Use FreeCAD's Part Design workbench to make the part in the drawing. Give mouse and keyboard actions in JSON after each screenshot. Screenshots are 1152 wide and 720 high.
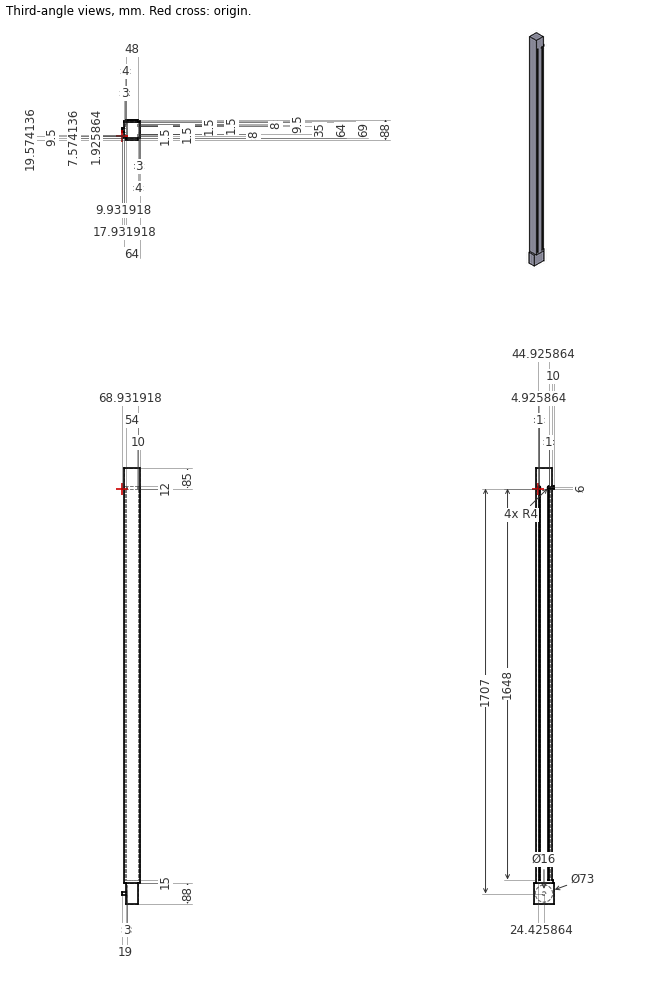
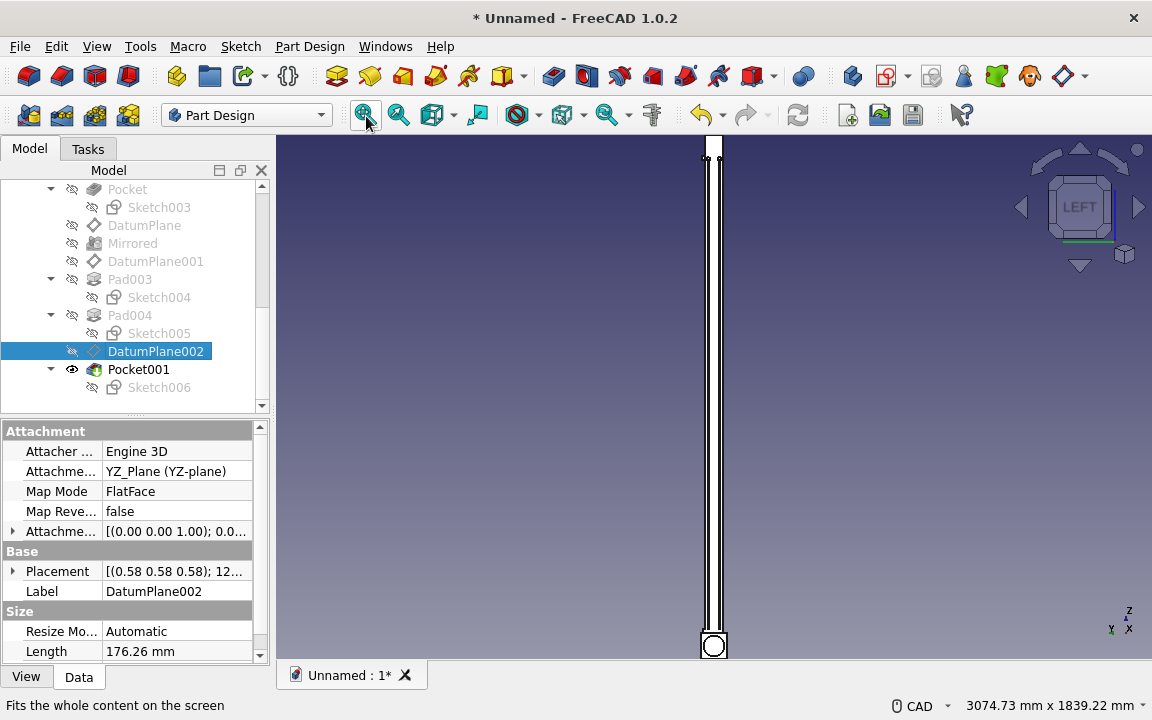
{"action": "left_click", "coordinate": [366, 116]}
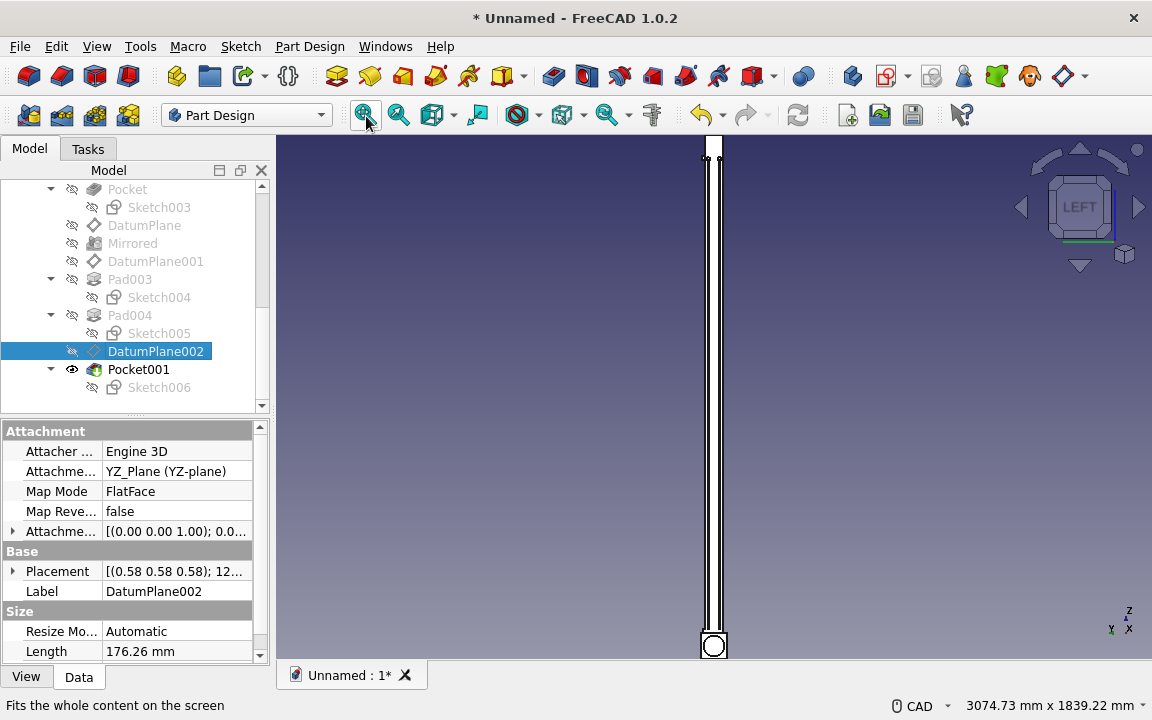
{"action": "key", "text": "2"}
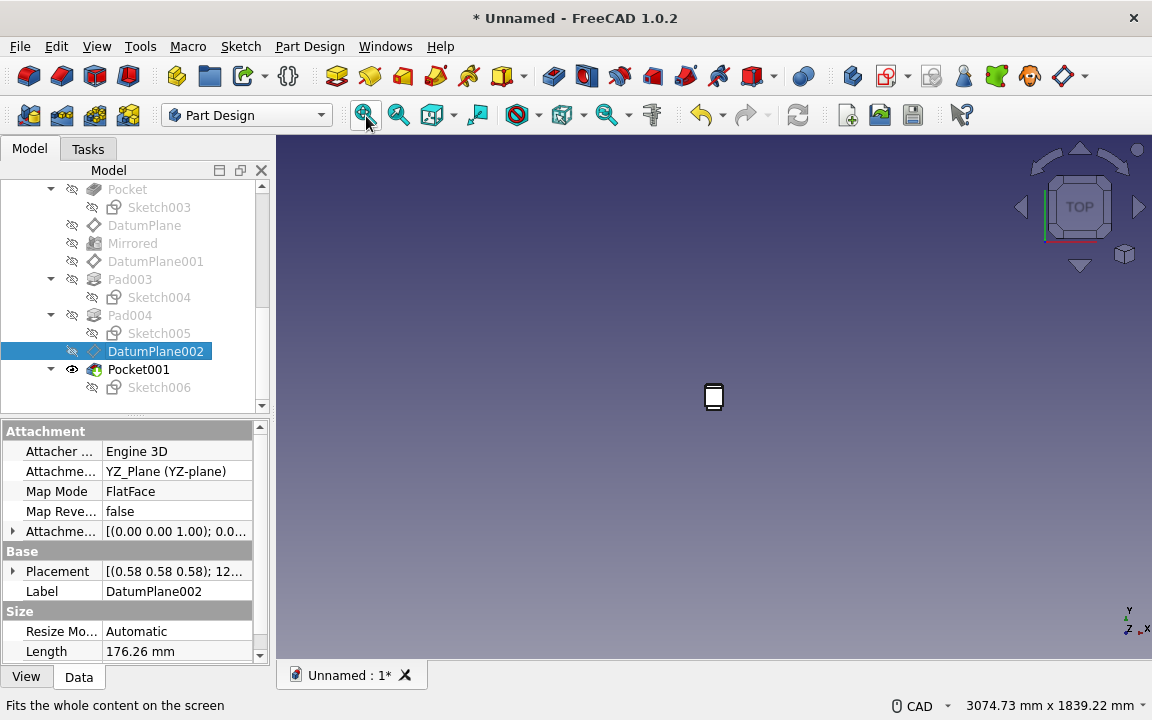
{"action": "left_click", "coordinate": [366, 116]}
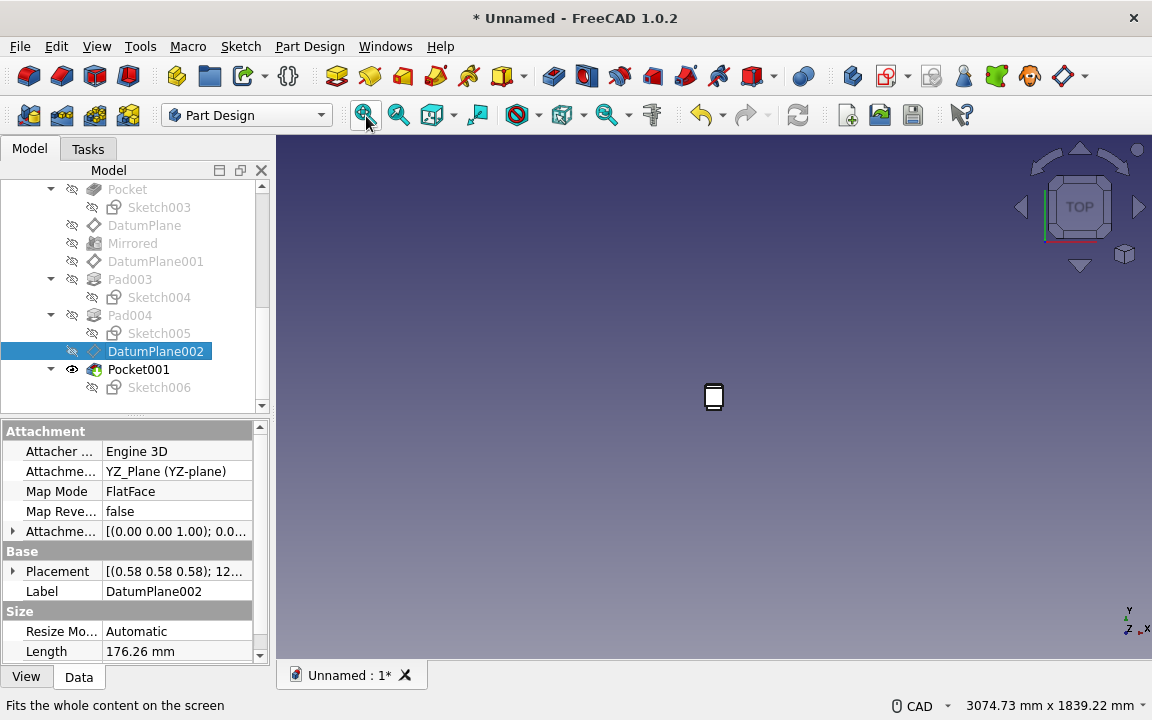
{"action": "key", "text": "1"}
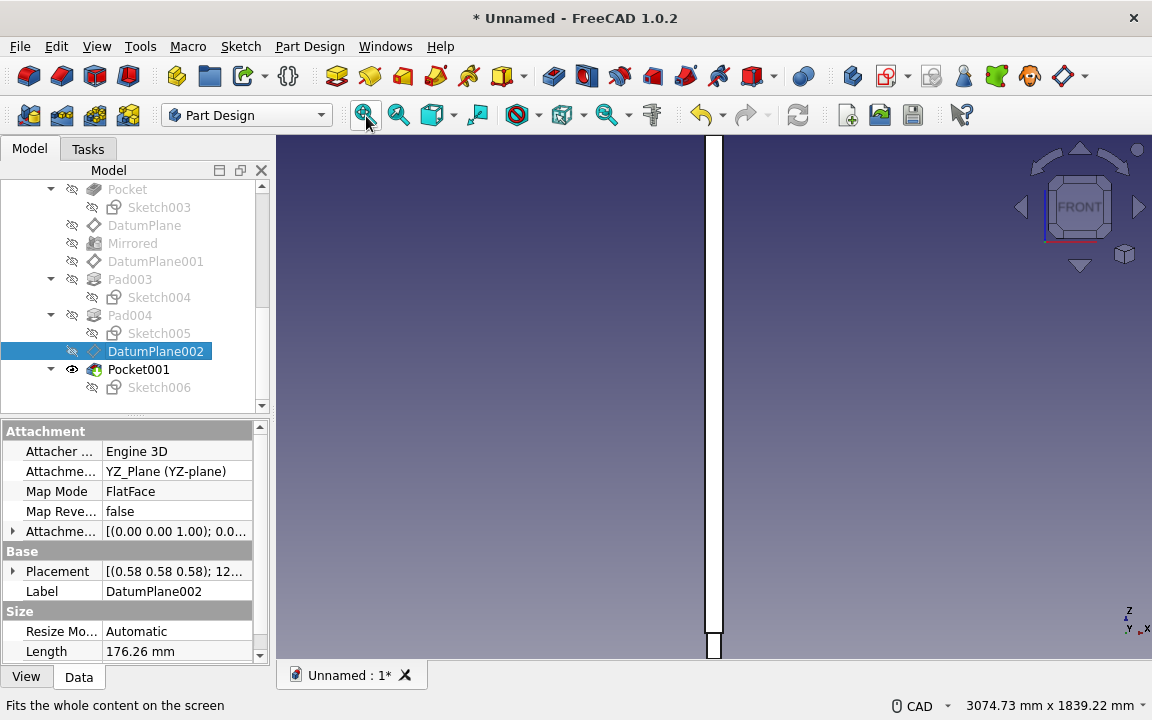
{"action": "left_click", "coordinate": [366, 116]}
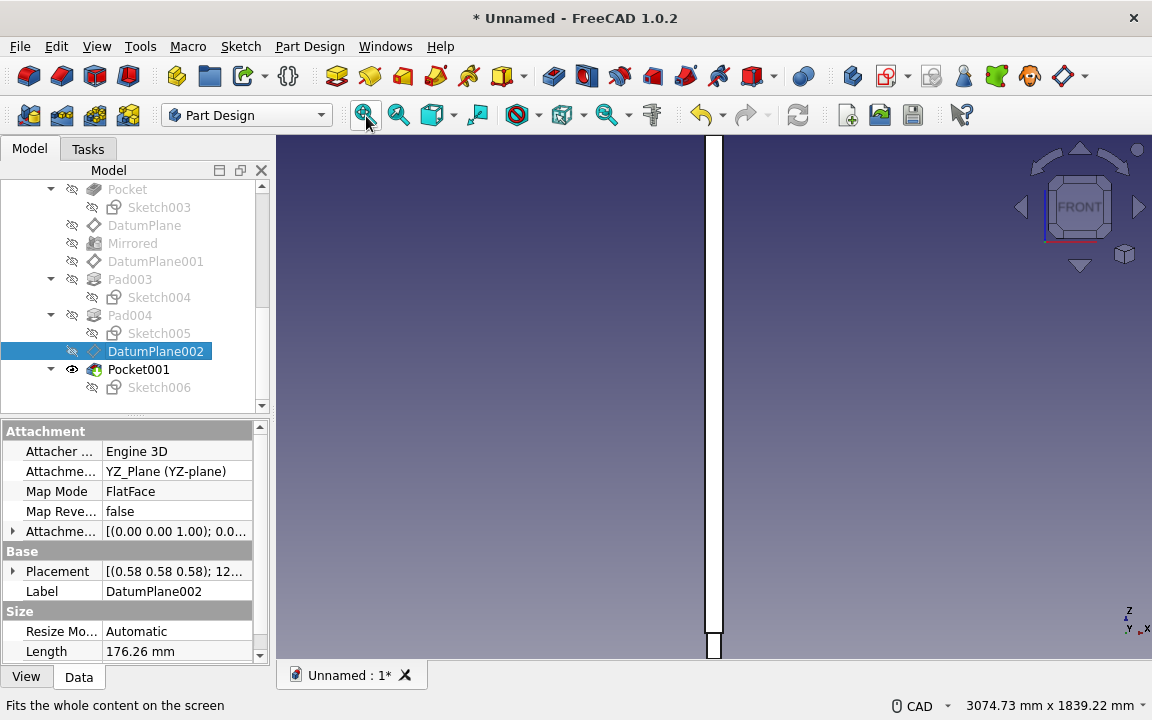
{"action": "scroll", "coordinate": [141, 293], "scroll_direction": "down", "scroll_amount": 3}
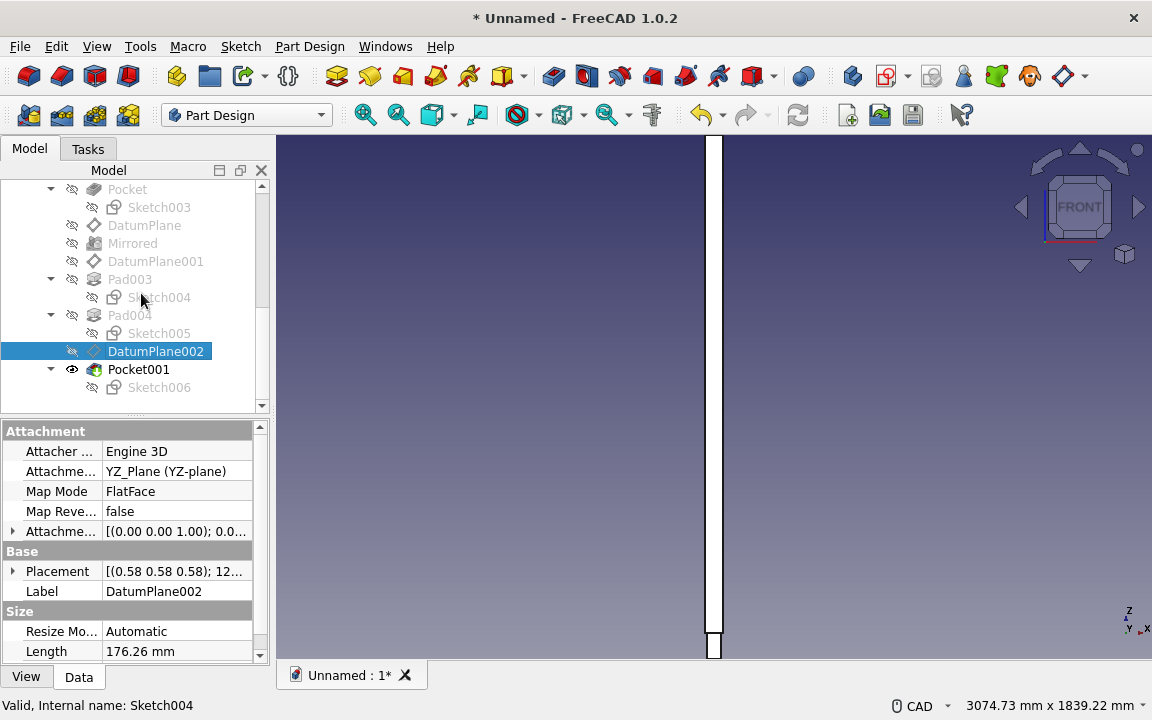
{"action": "scroll", "coordinate": [141, 293], "scroll_direction": "up", "scroll_amount": 15}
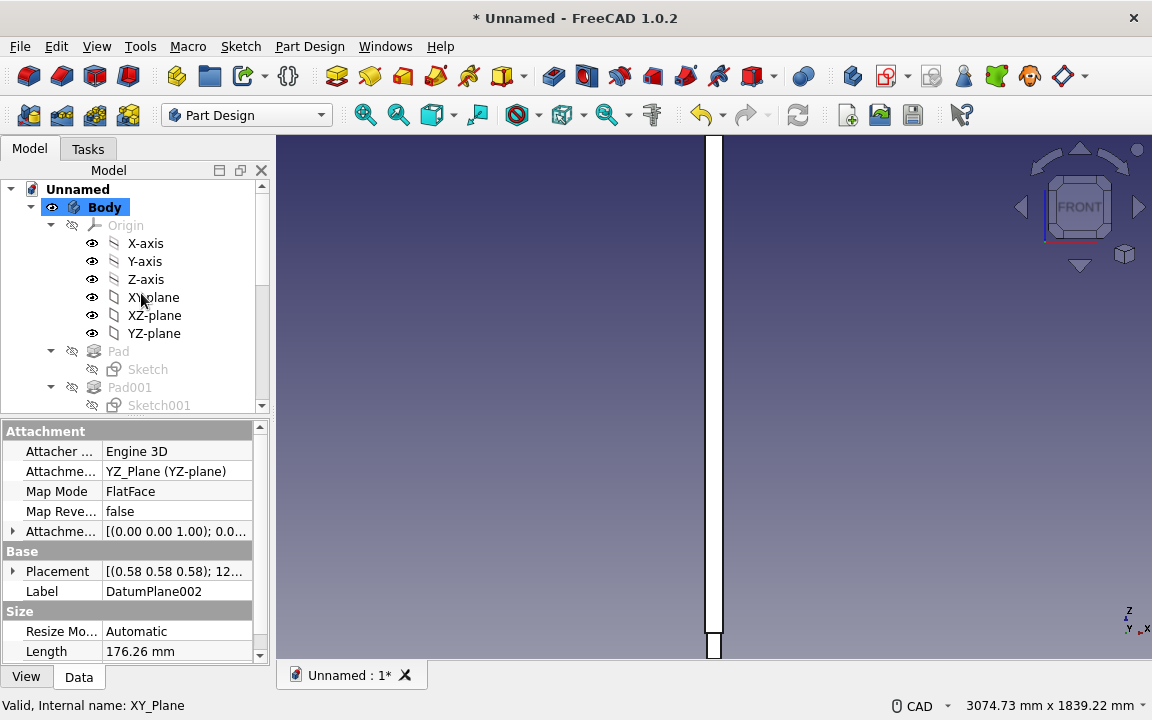
{"action": "left_click", "coordinate": [137, 333]}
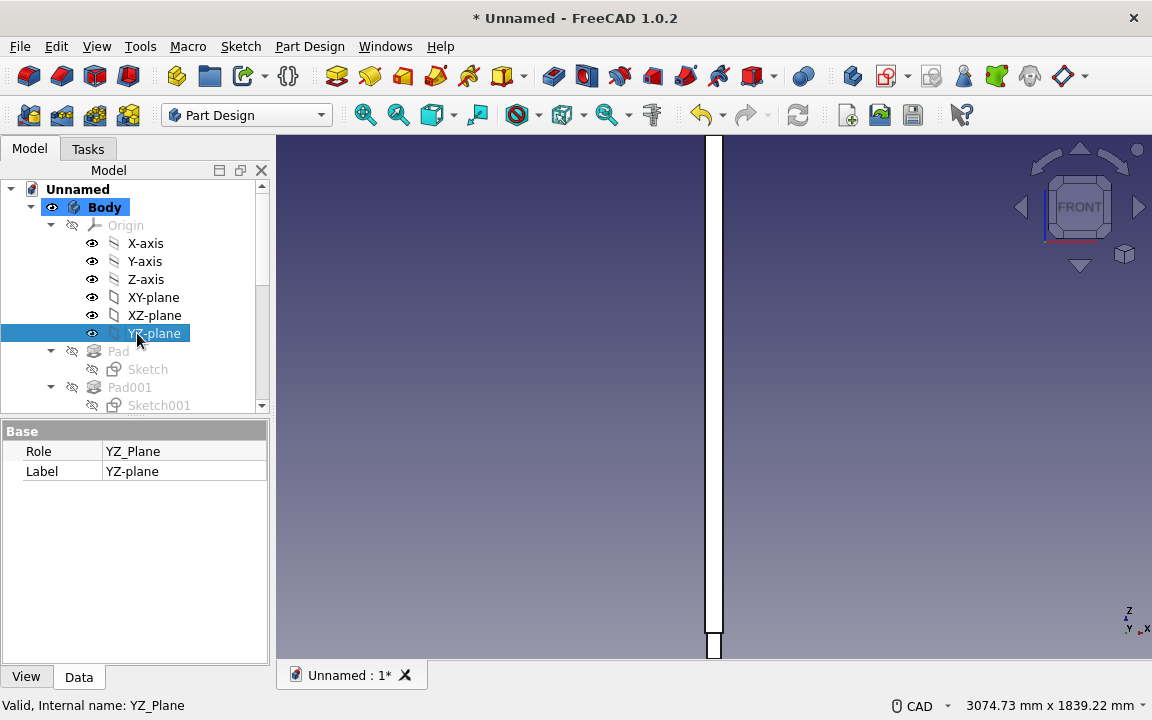
{"action": "left_click", "coordinate": [1062, 76]}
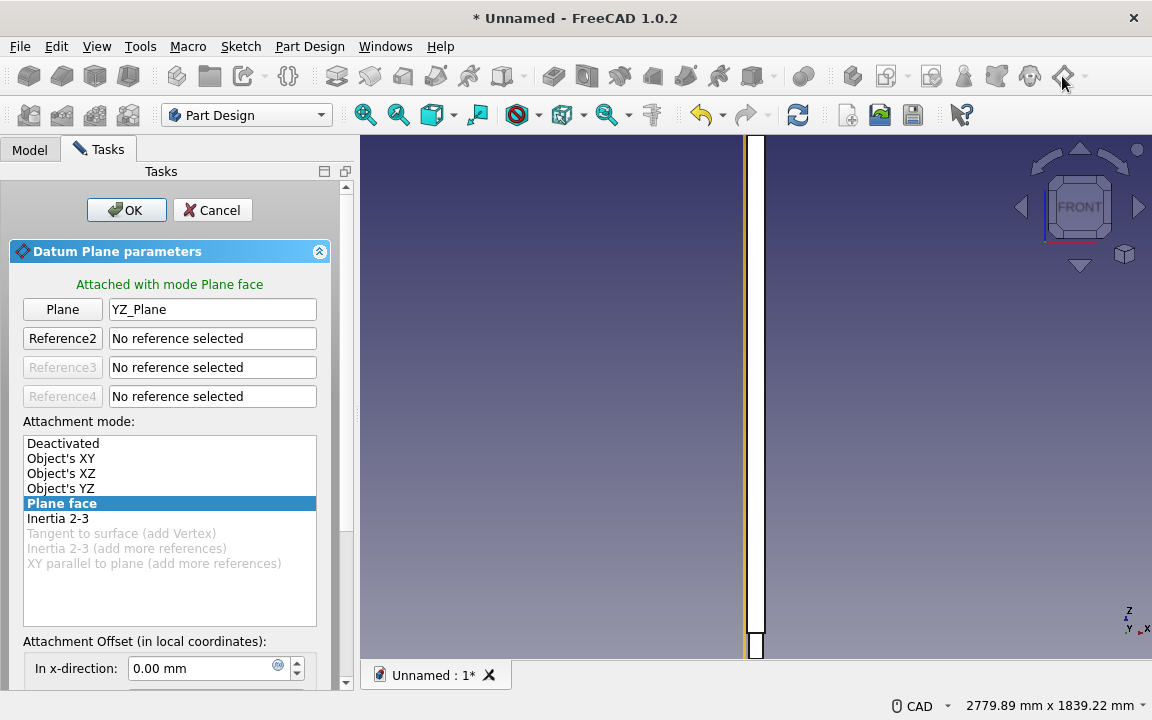
{"action": "scroll", "coordinate": [346, 436], "scroll_direction": "down", "scroll_amount": 2}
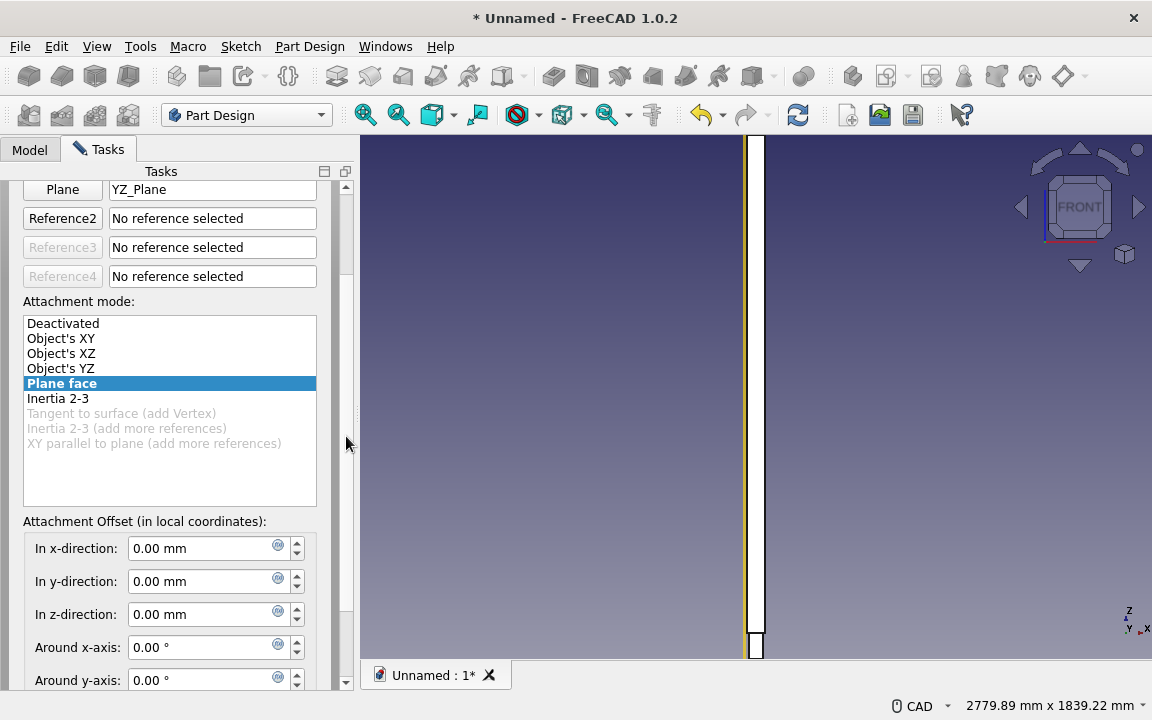
{"action": "triple_click", "coordinate": [210, 614]}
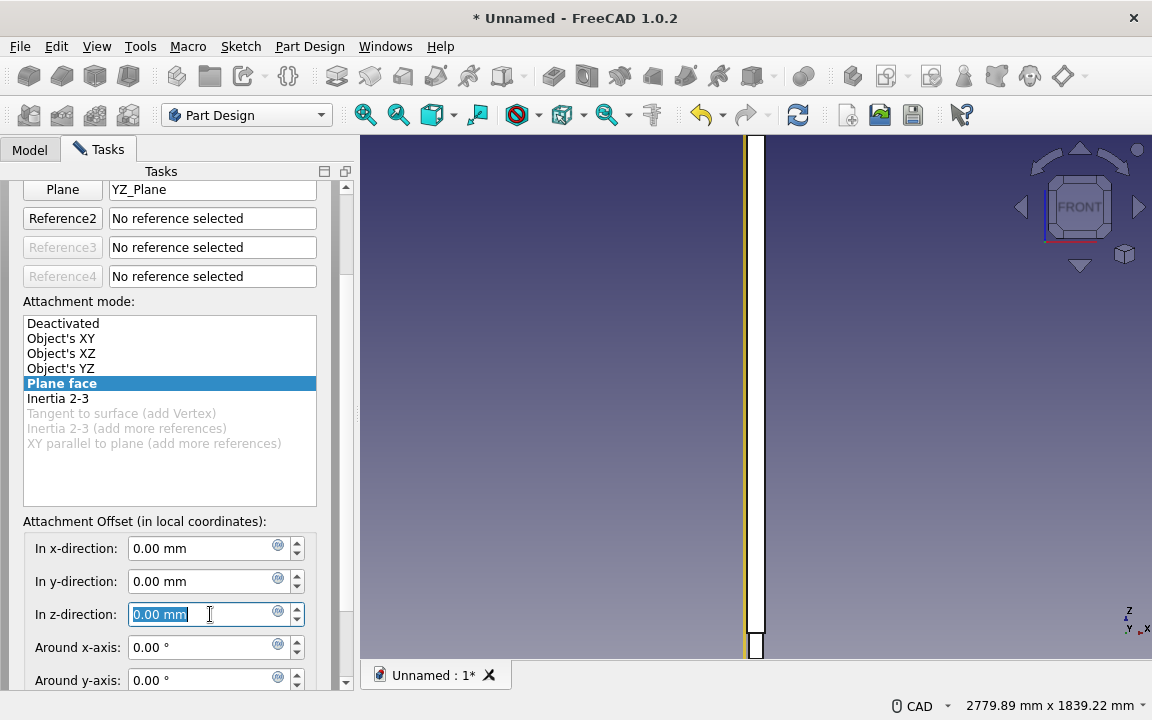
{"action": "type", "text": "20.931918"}
{"action": "key", "text": "Tab"}